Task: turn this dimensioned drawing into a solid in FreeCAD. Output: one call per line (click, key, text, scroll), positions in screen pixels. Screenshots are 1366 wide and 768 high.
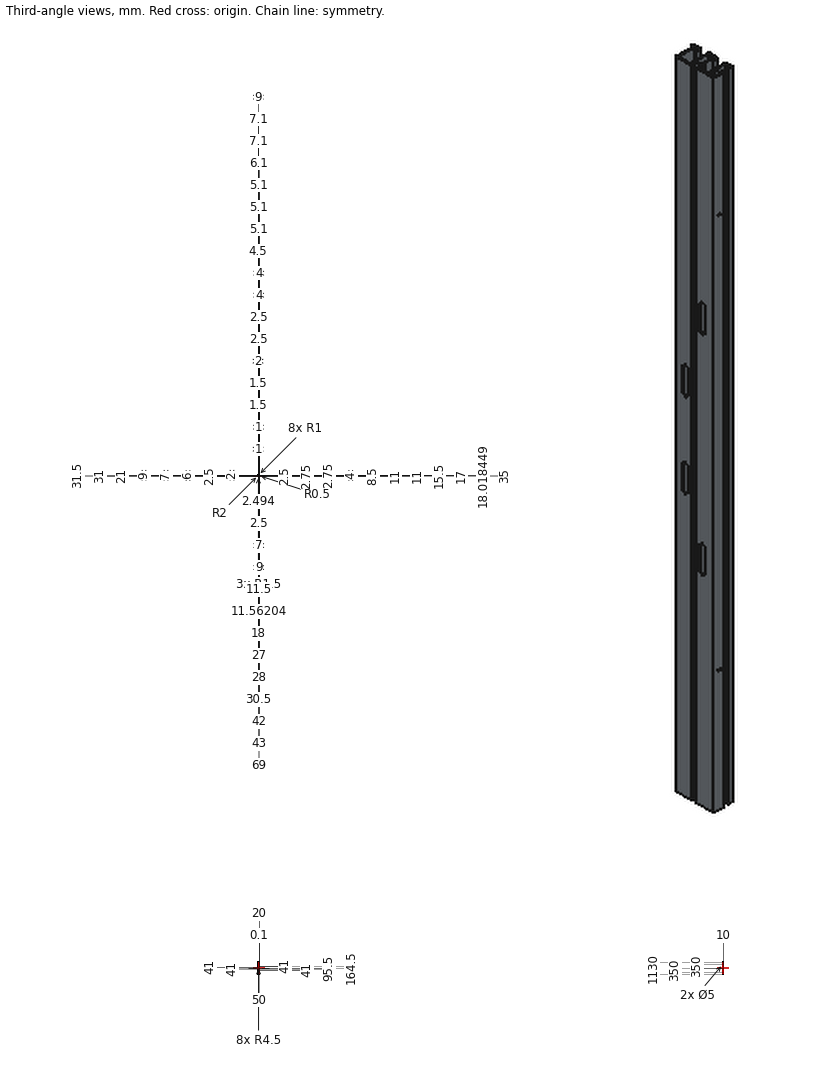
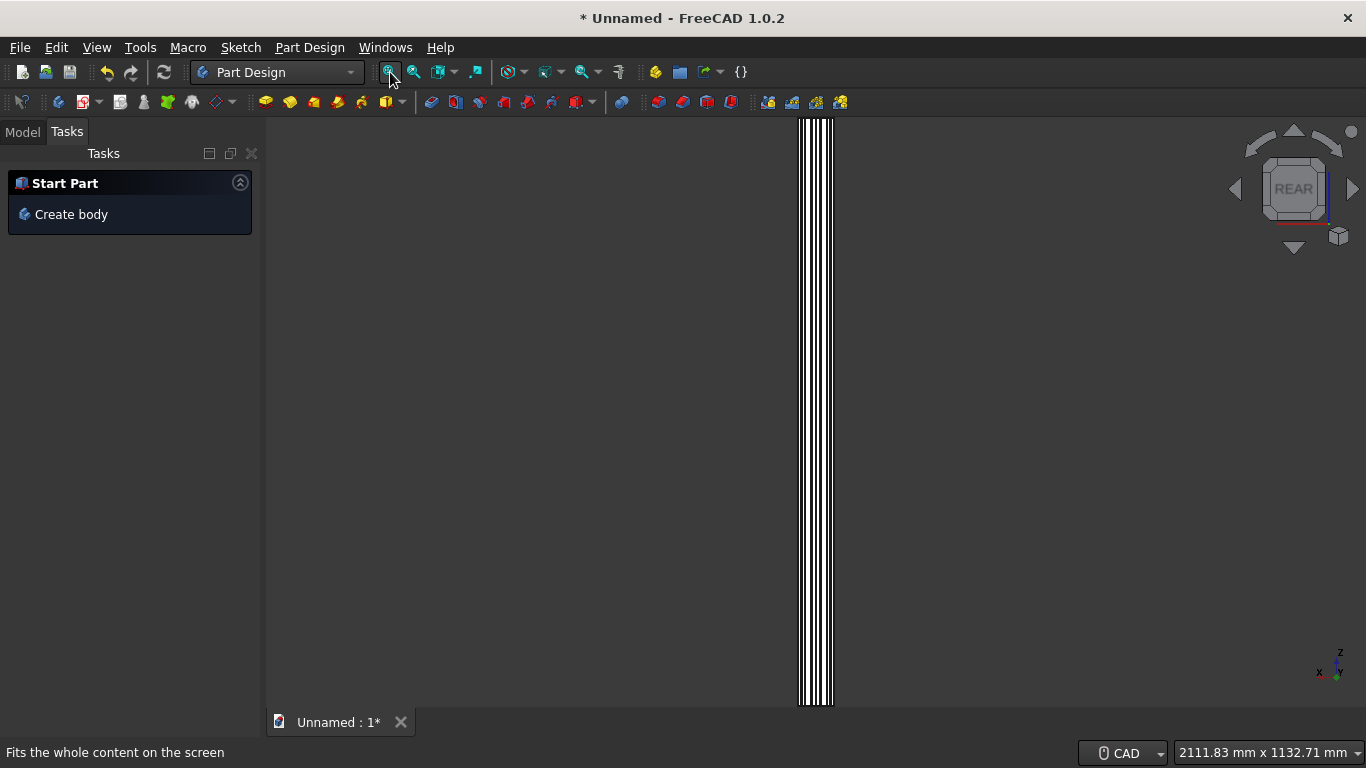
key(2)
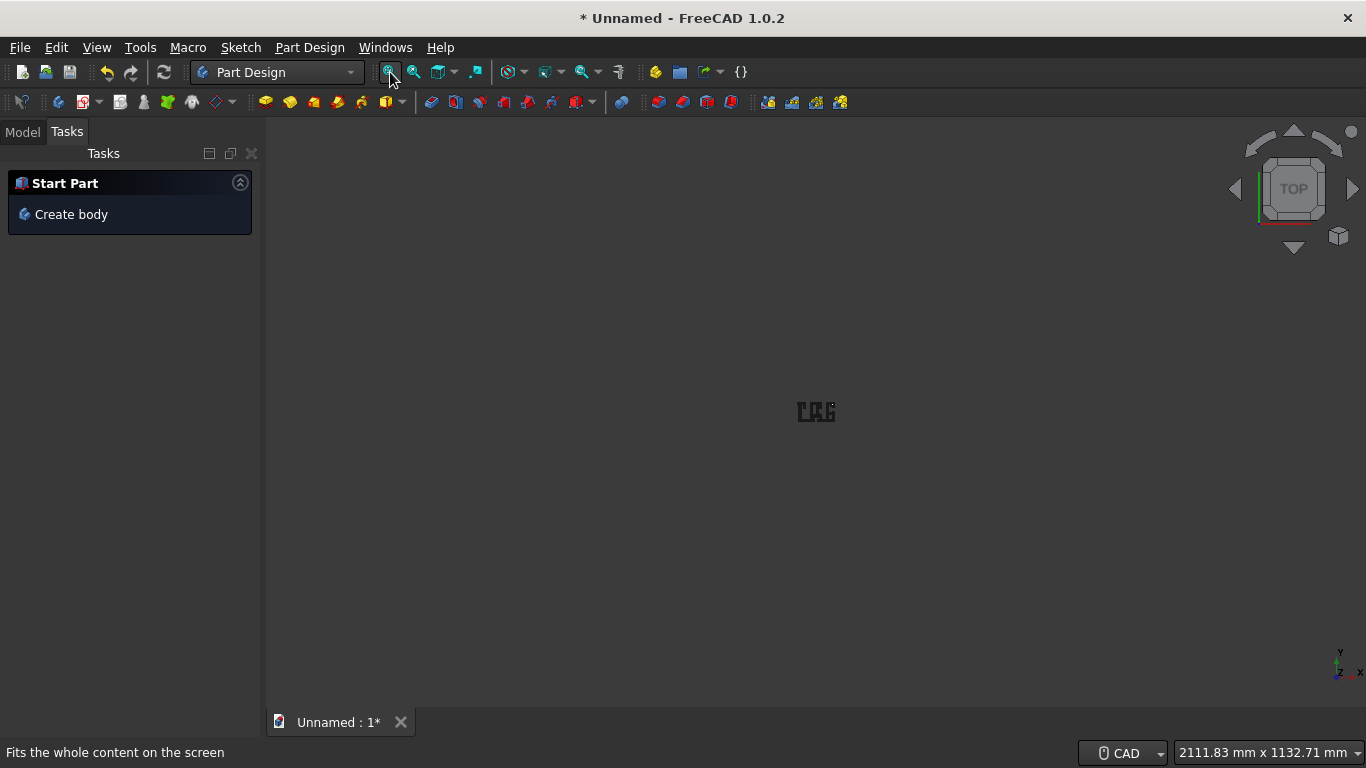
click(390, 72)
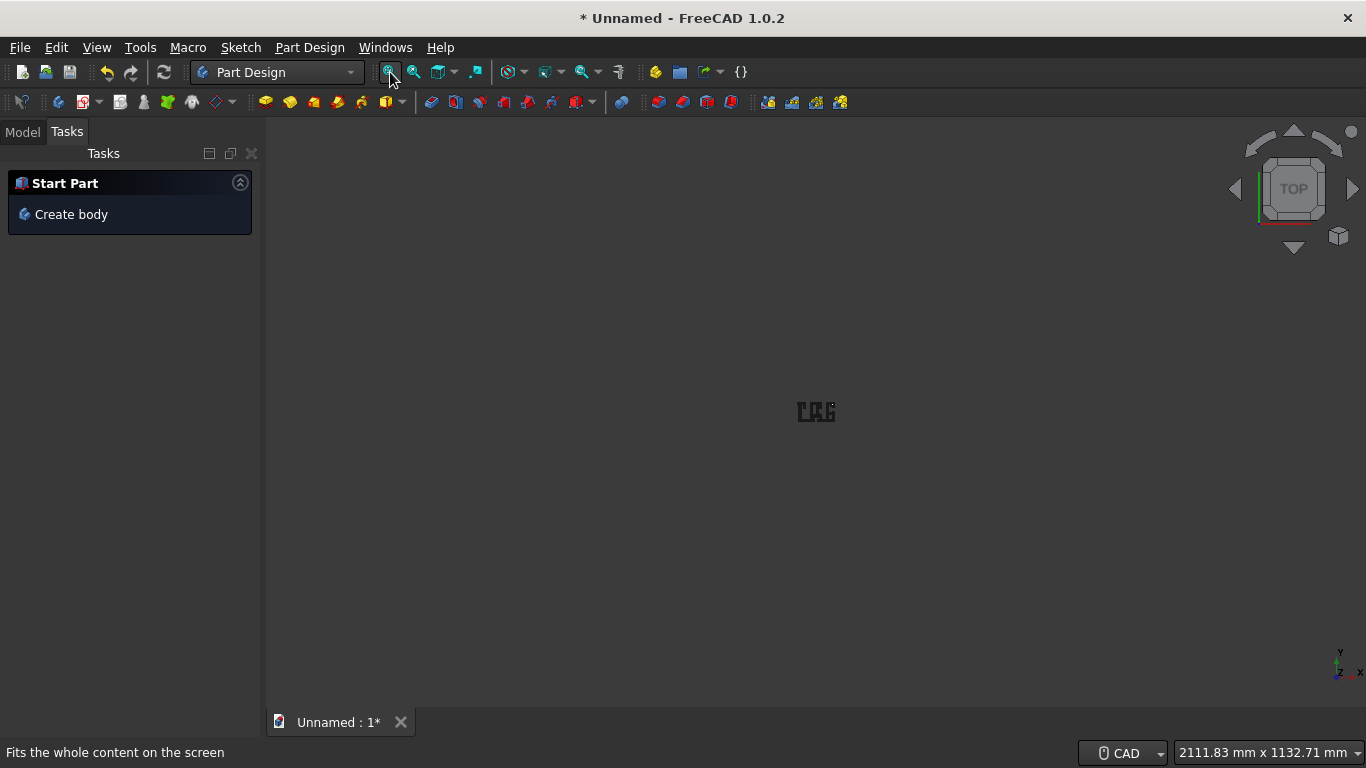
key(3)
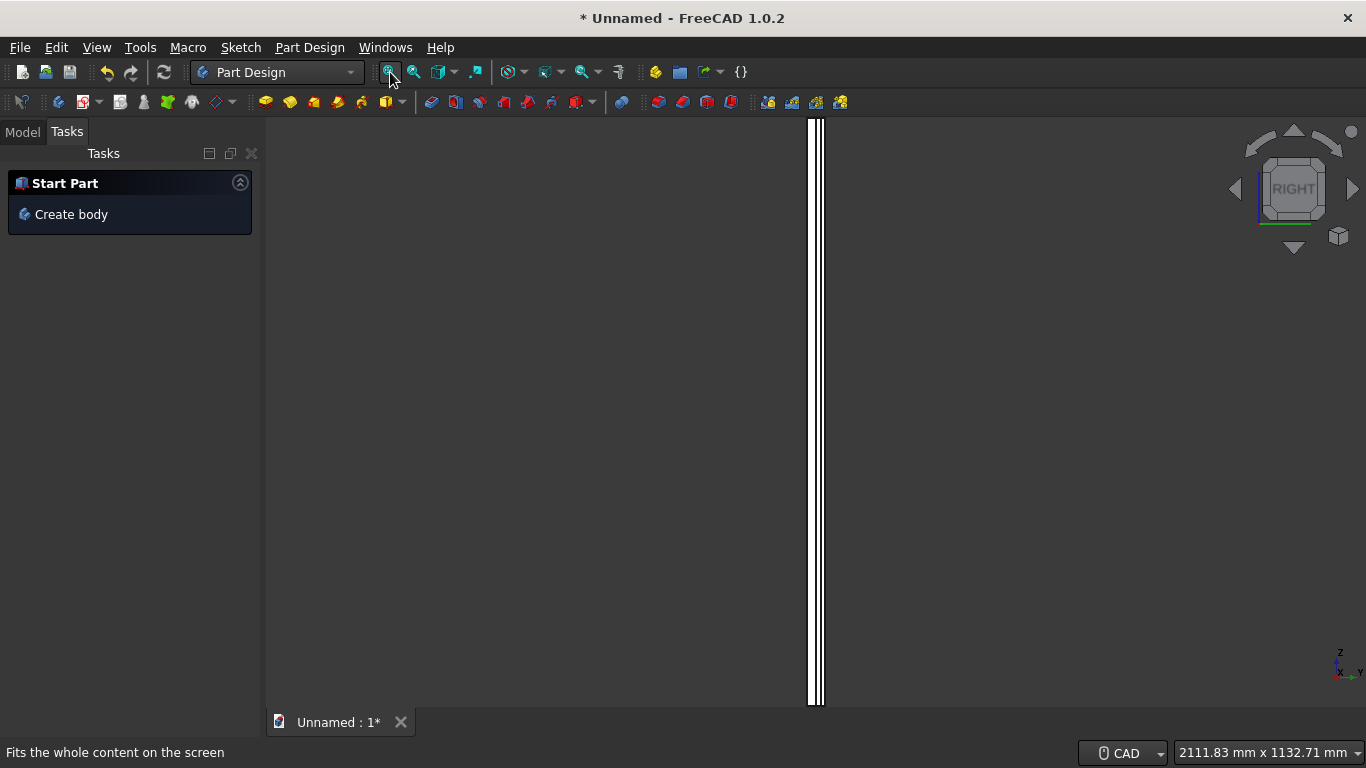
click(23, 131)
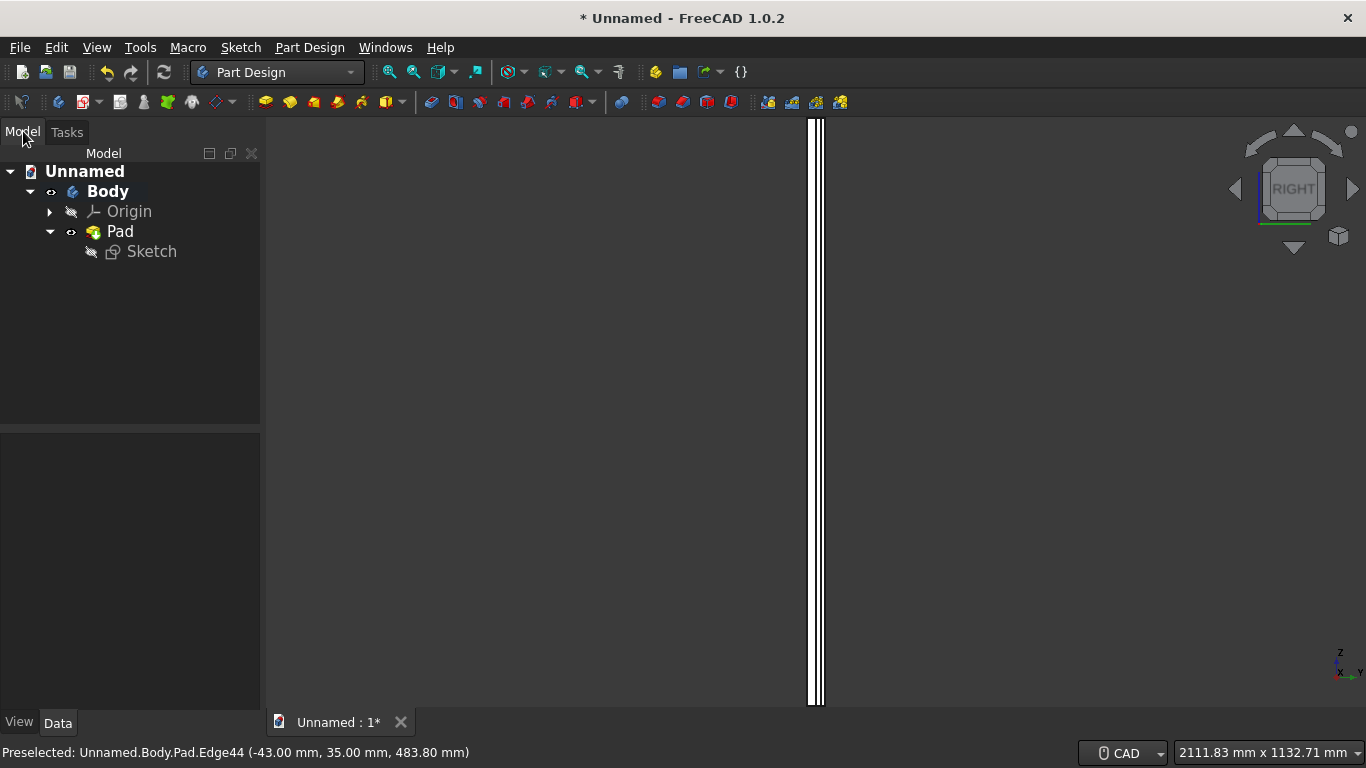
click(50, 212)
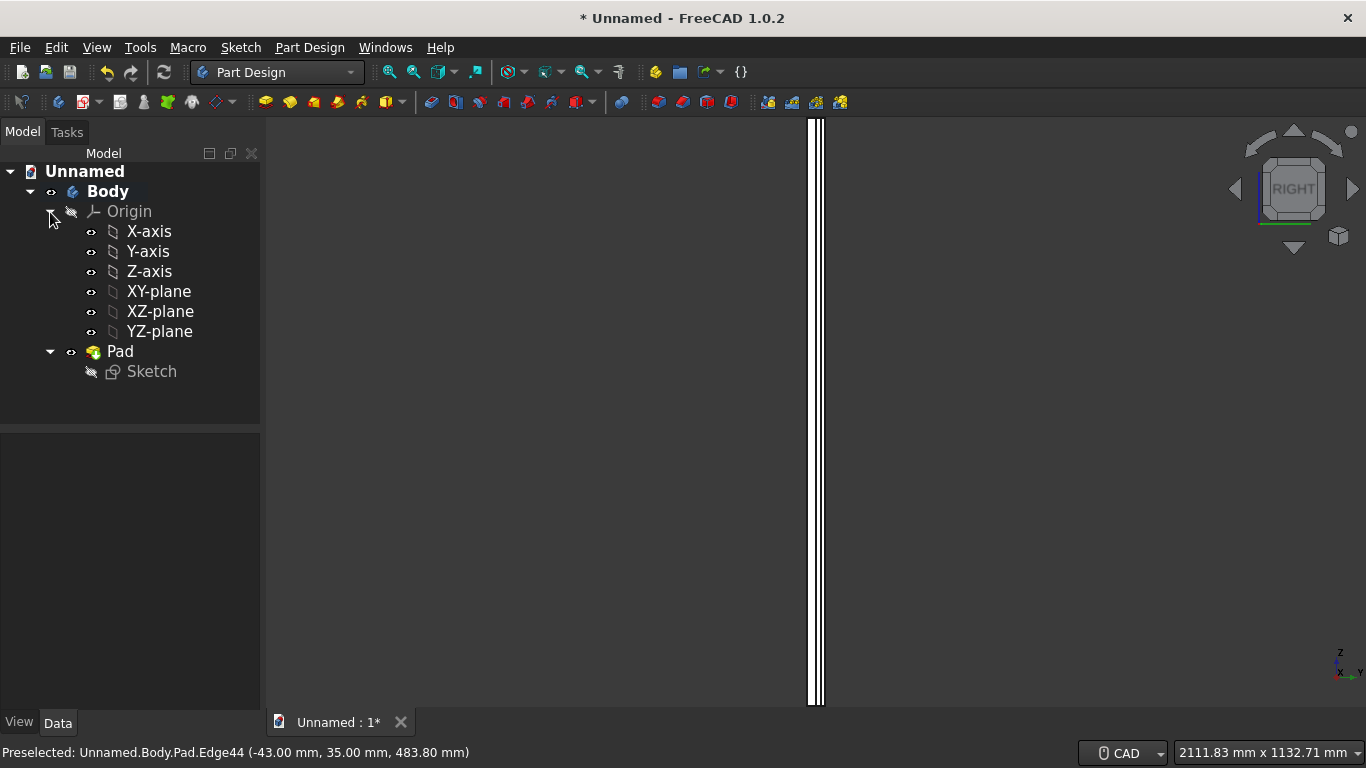
click(136, 312)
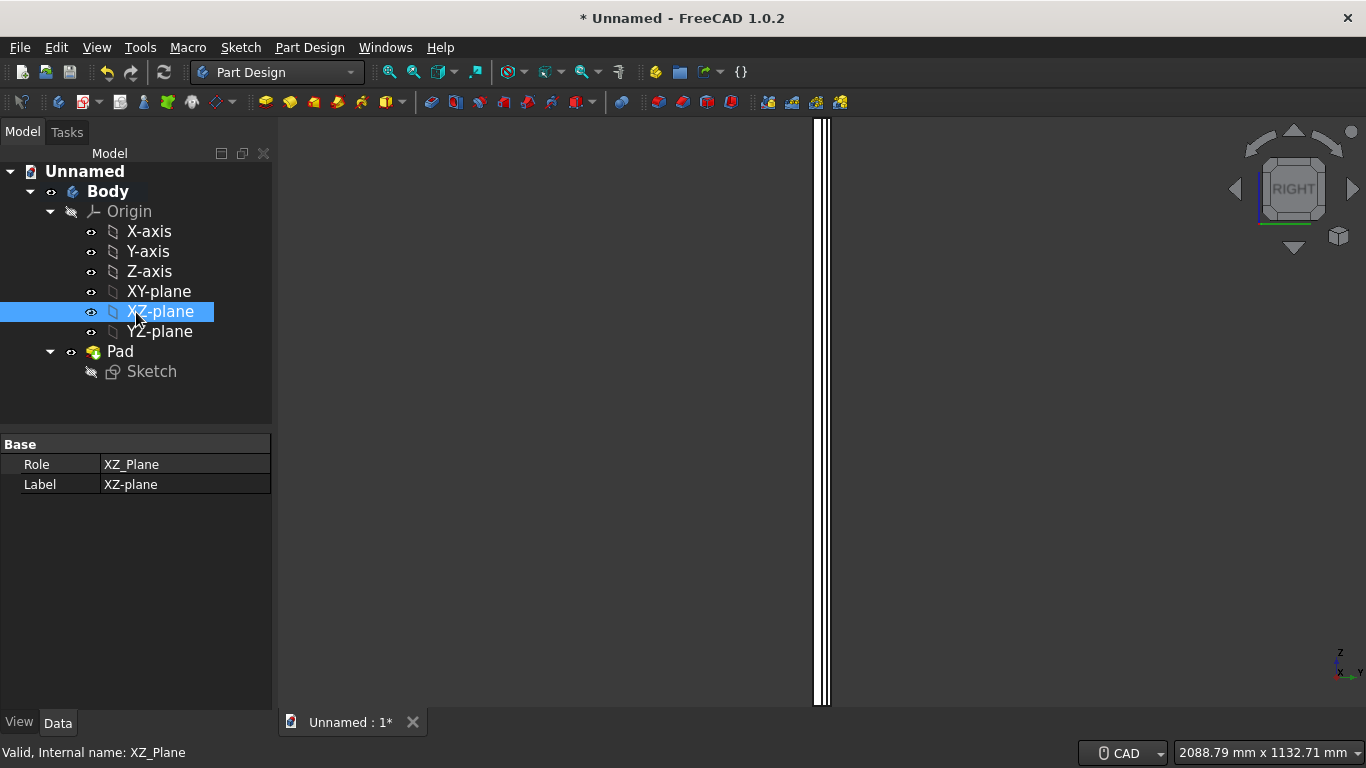
click(216, 102)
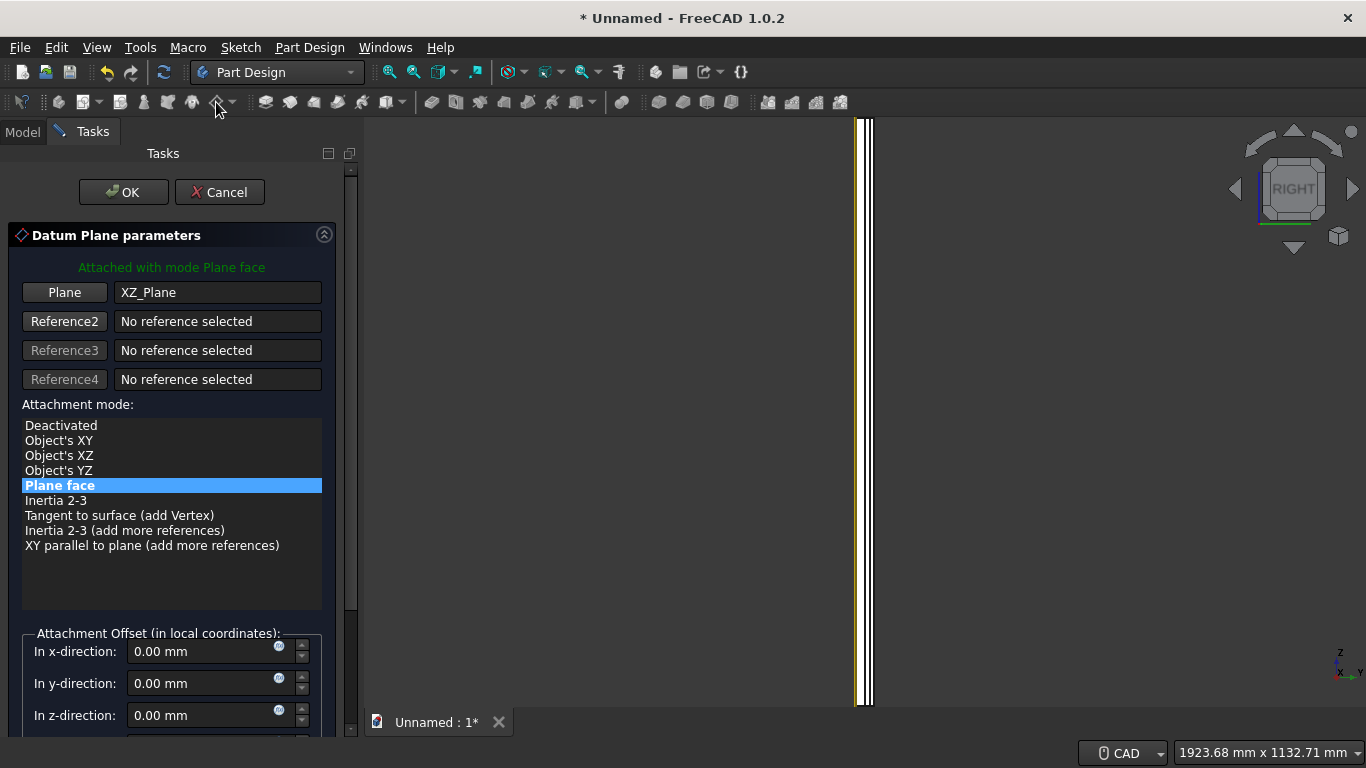
triple_click(210, 715)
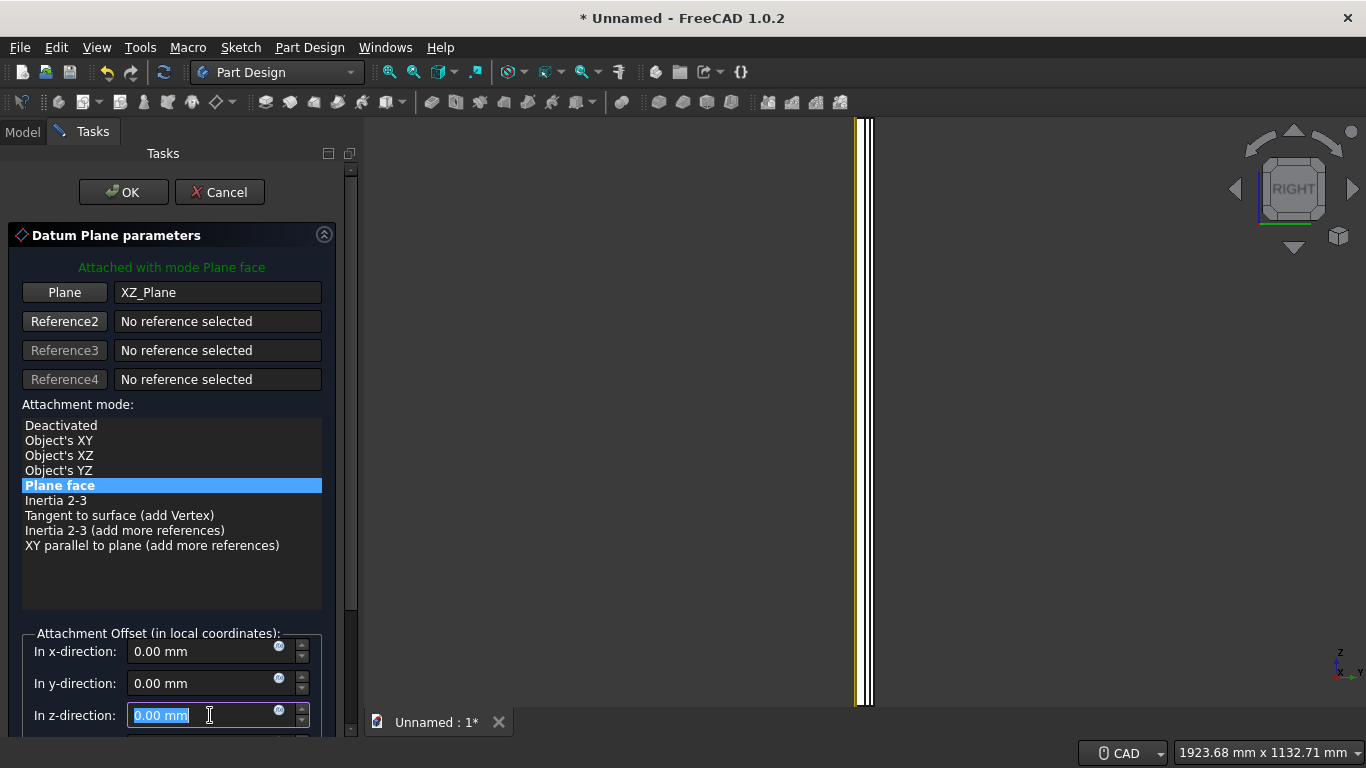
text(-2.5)
key(Tab)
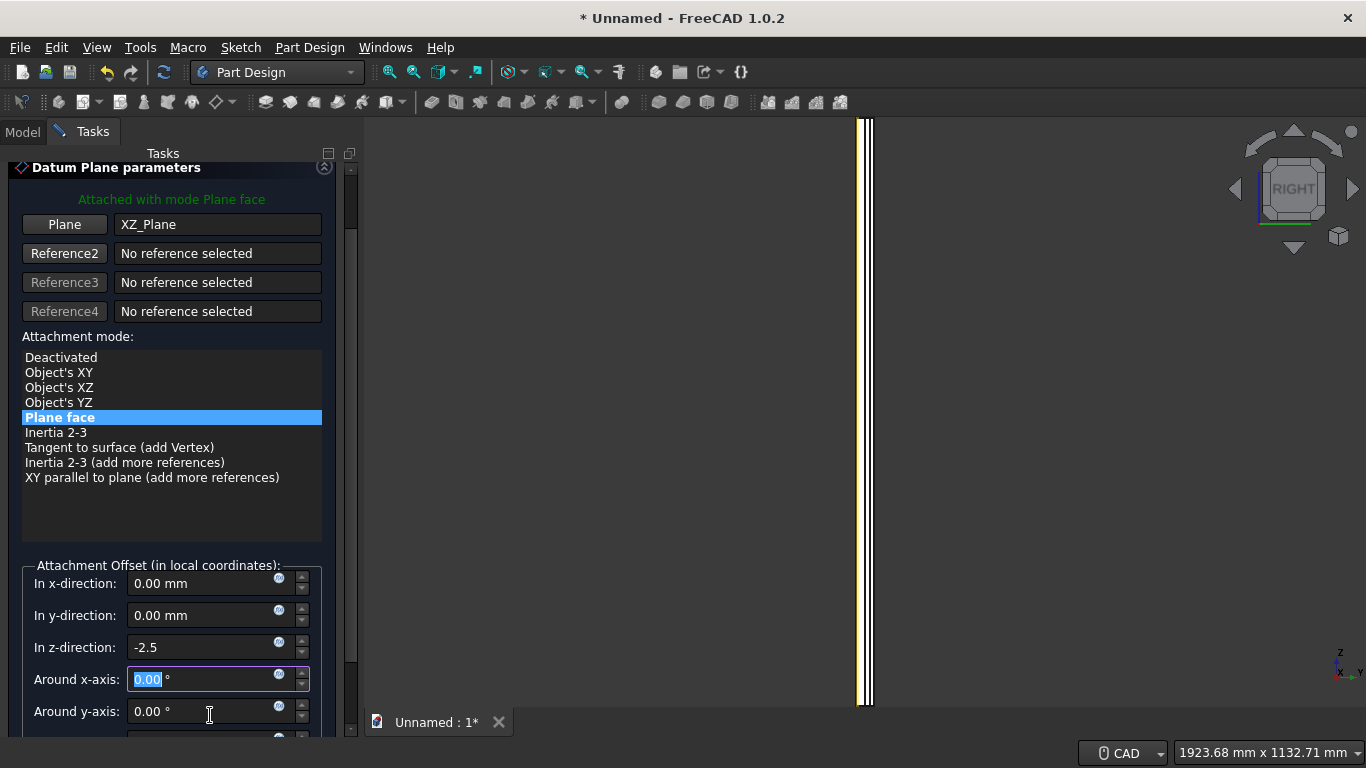
scroll(351, 450, up, 2)